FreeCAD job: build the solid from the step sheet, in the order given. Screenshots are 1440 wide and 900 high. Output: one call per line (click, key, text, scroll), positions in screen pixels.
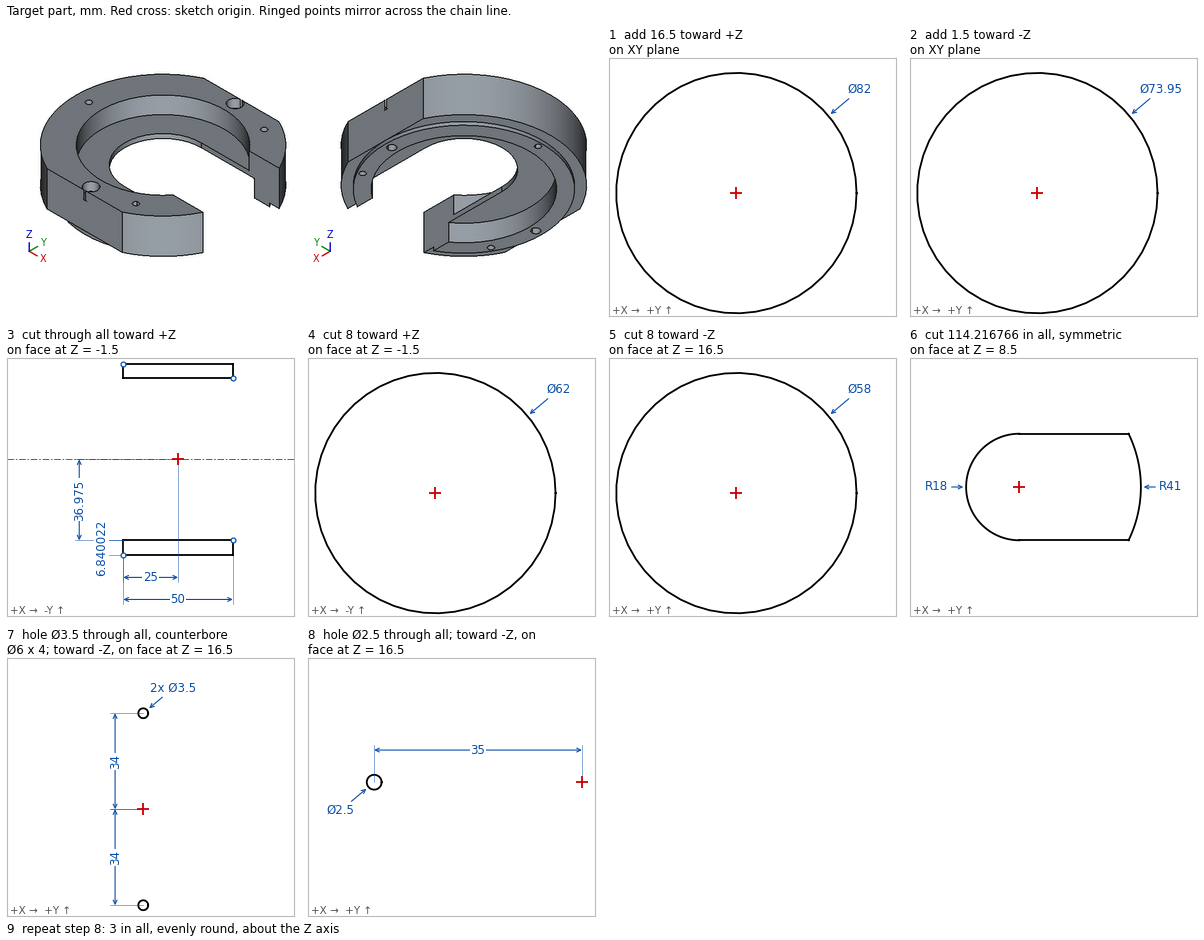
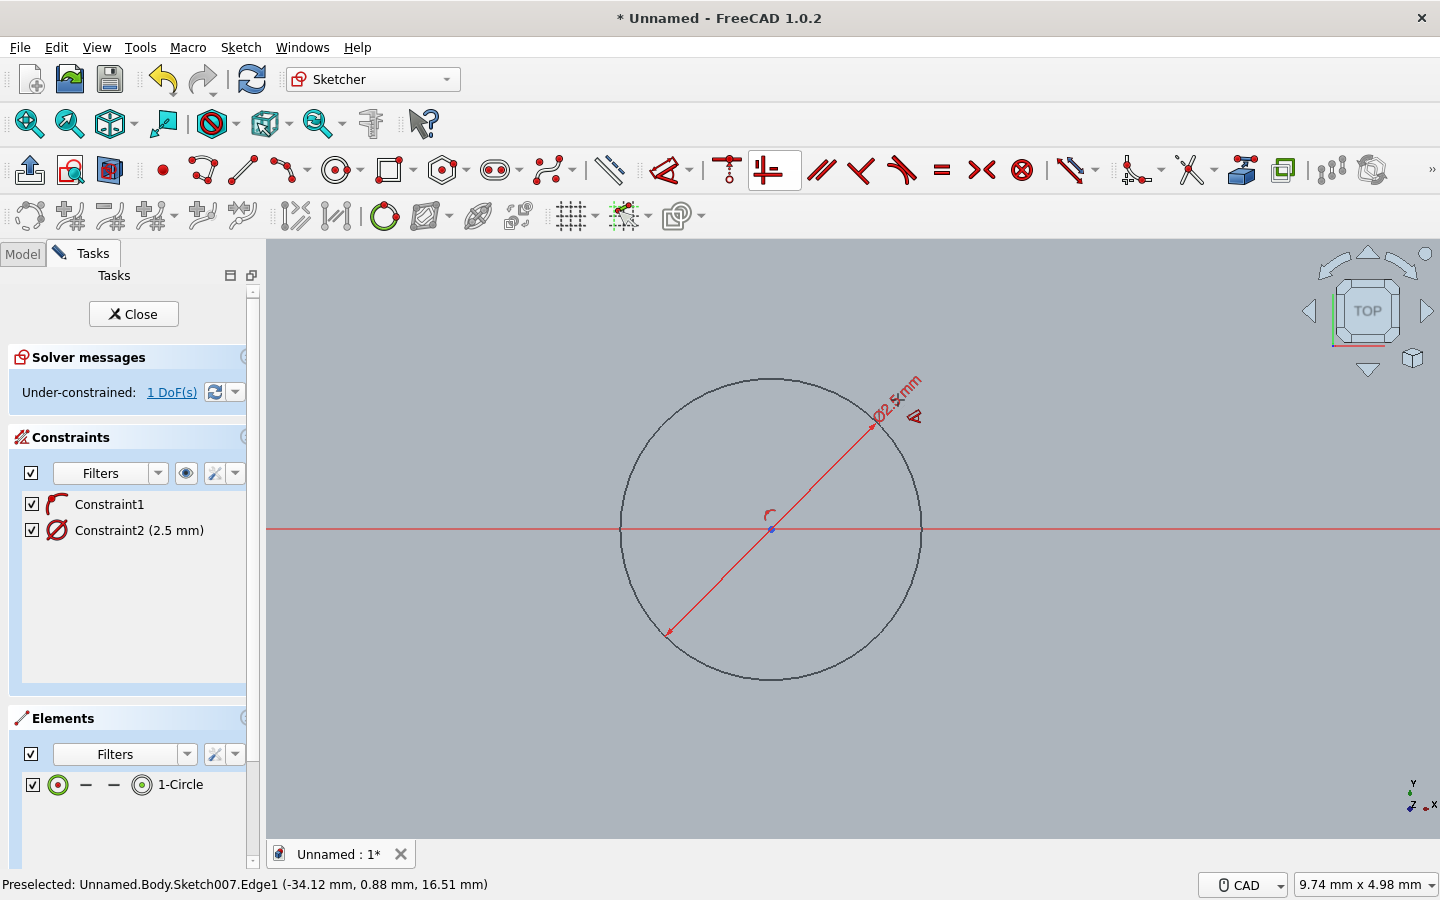
click(771, 529)
click(1023, 563)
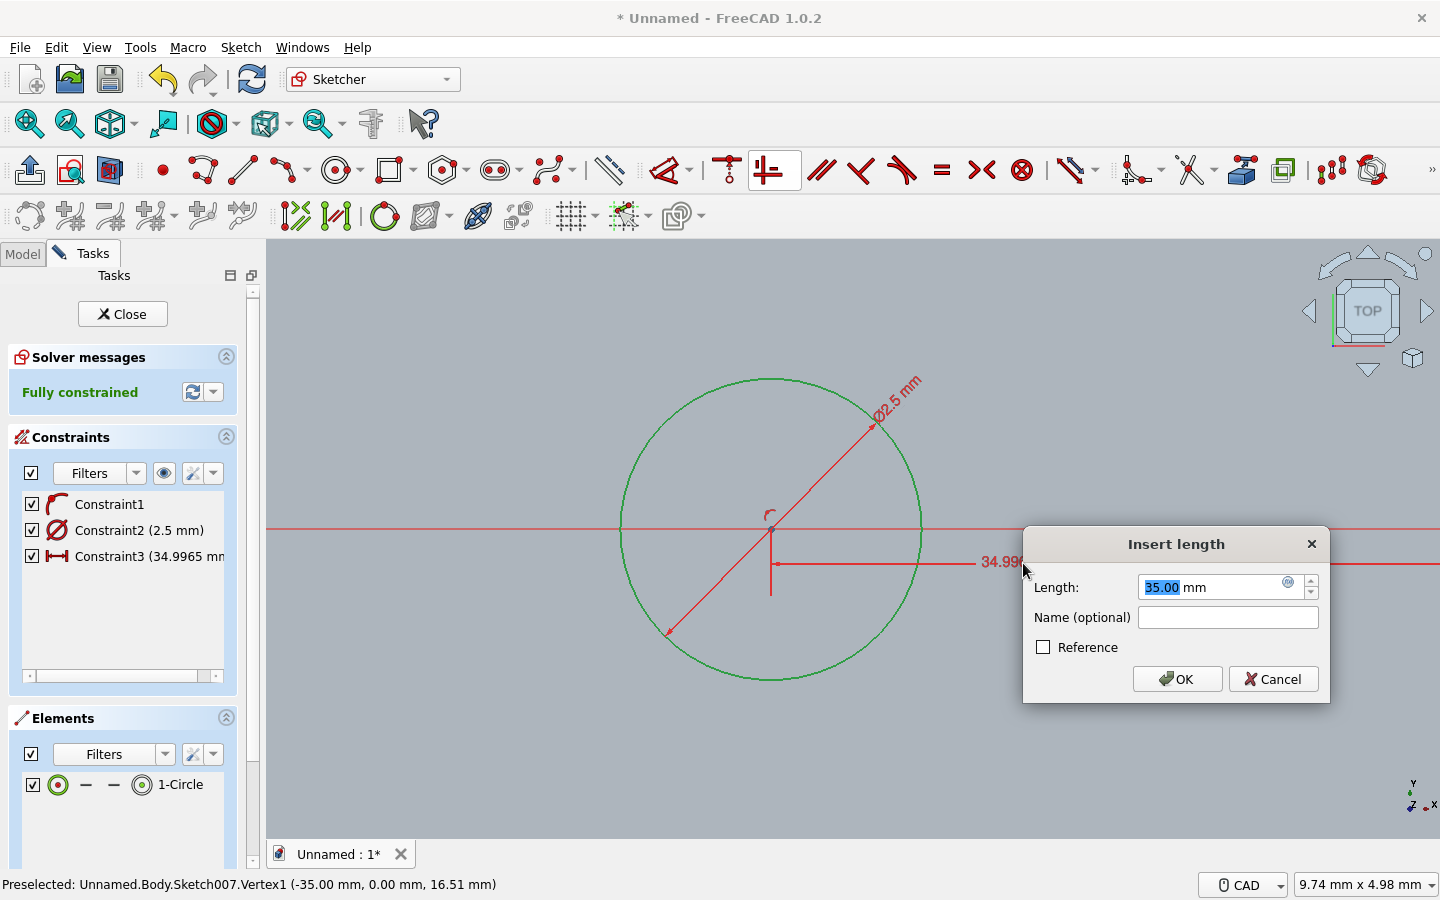
text(35)
key(Return)
key(Escape)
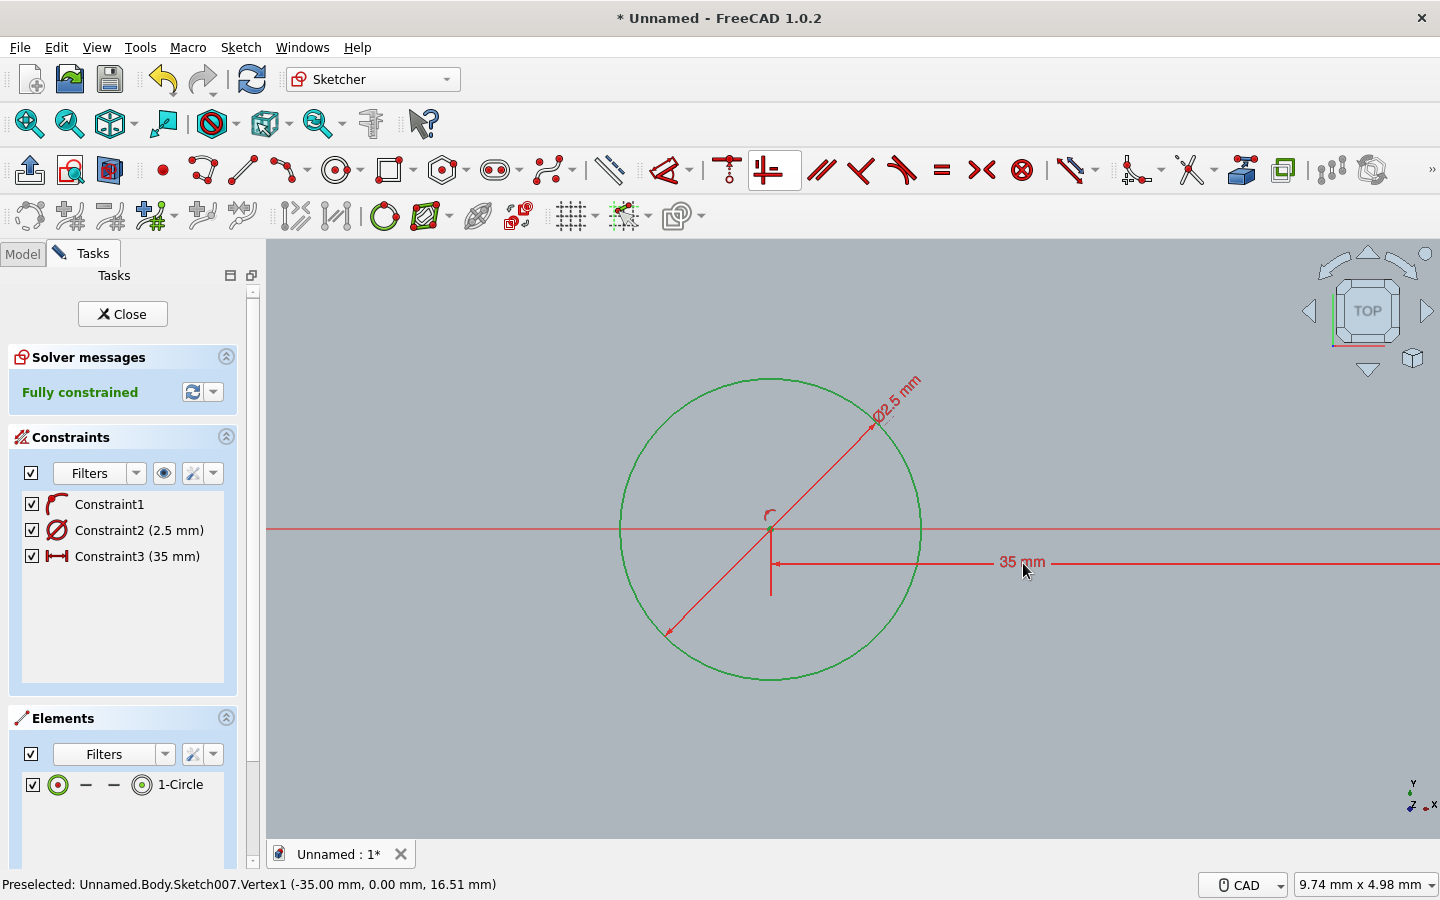
click(123, 314)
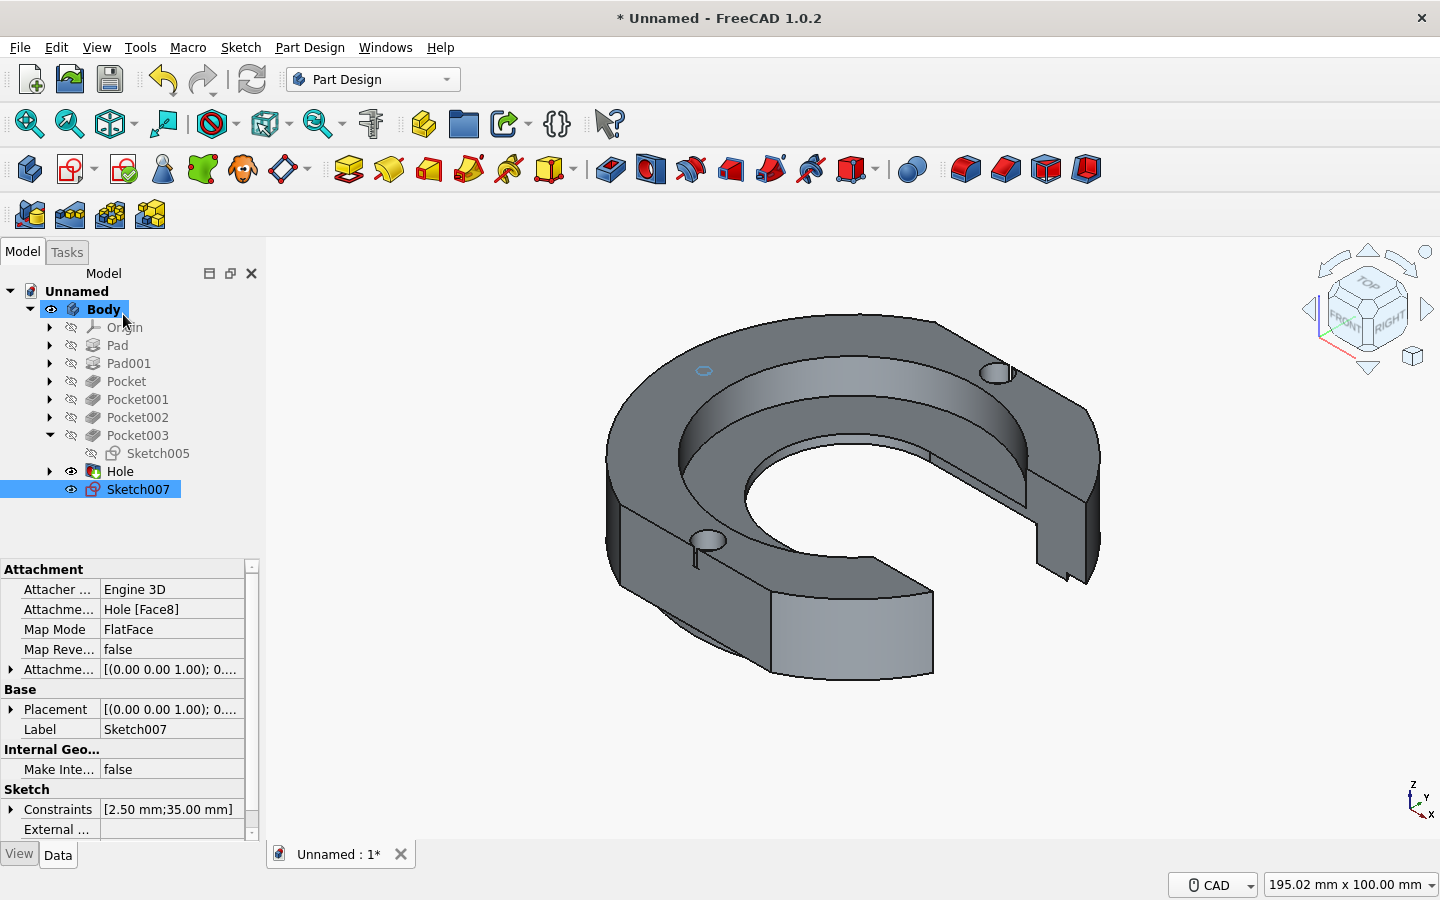
click(652, 170)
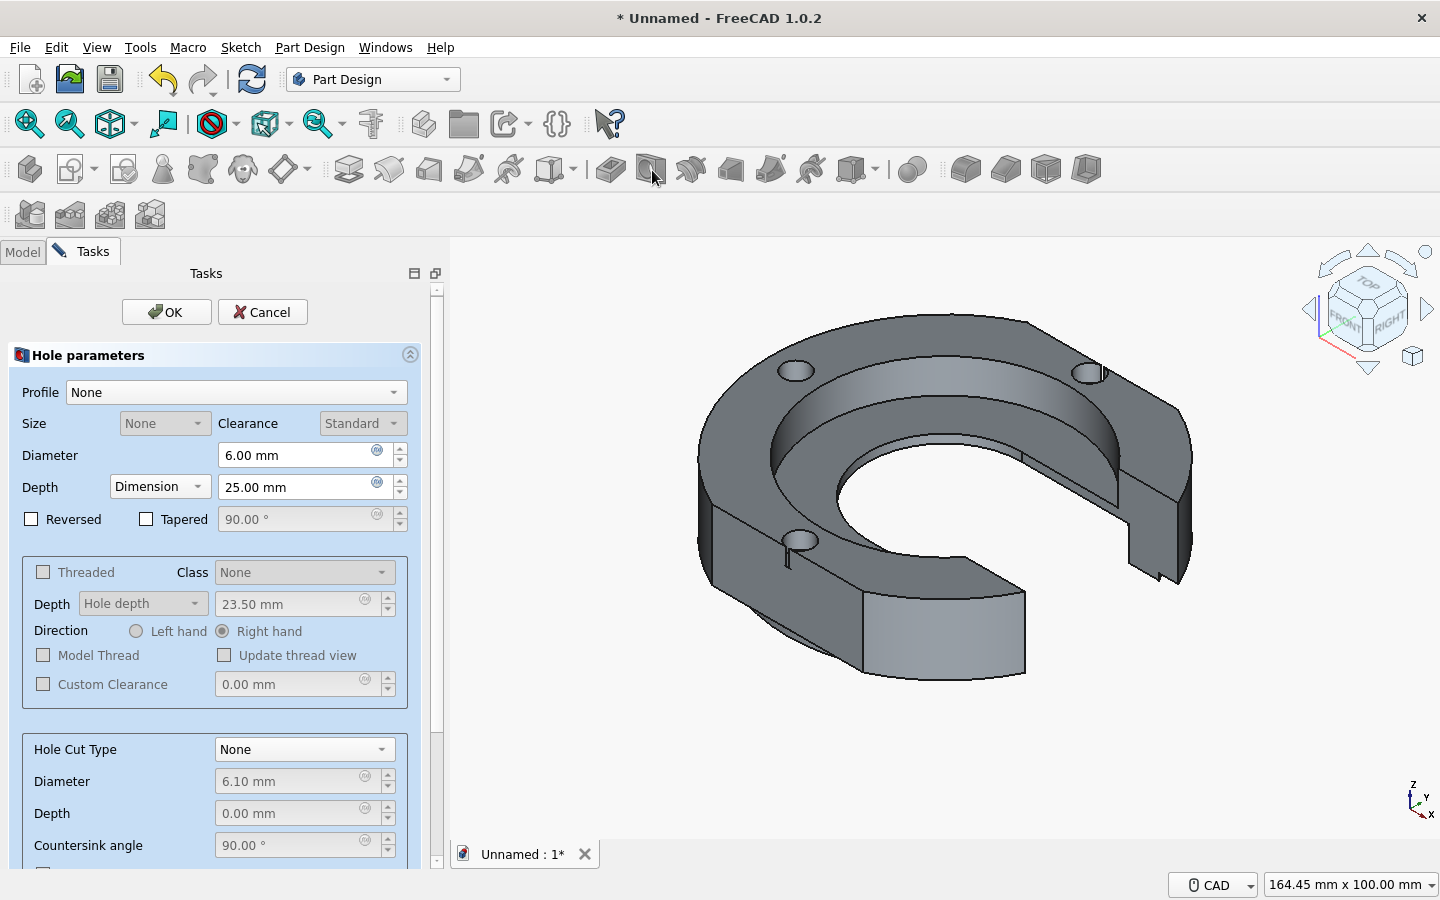
triple_click(305, 455)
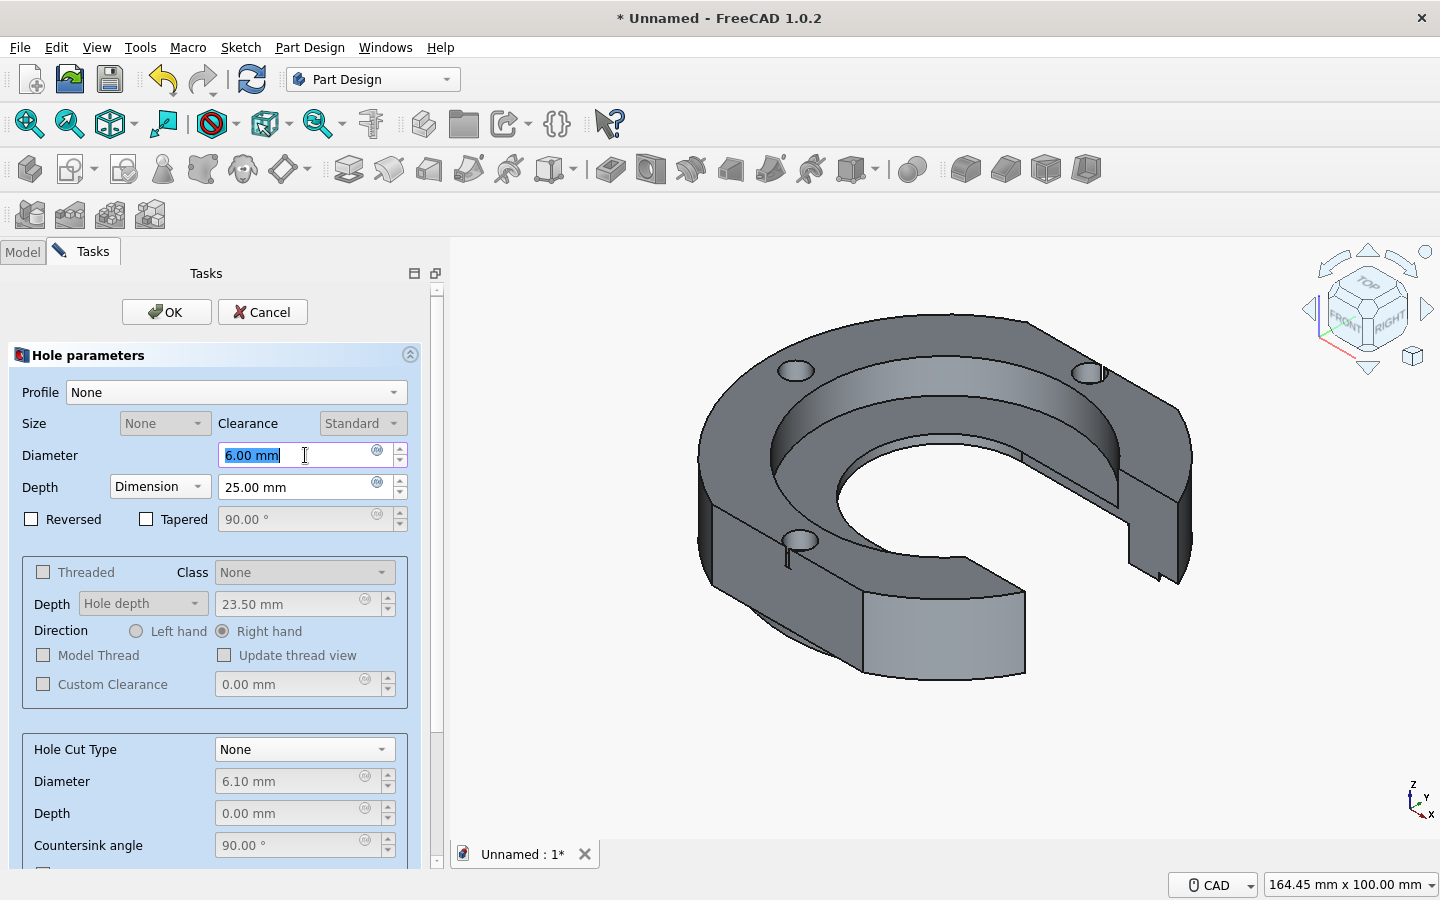
text(2.5)
key(Tab)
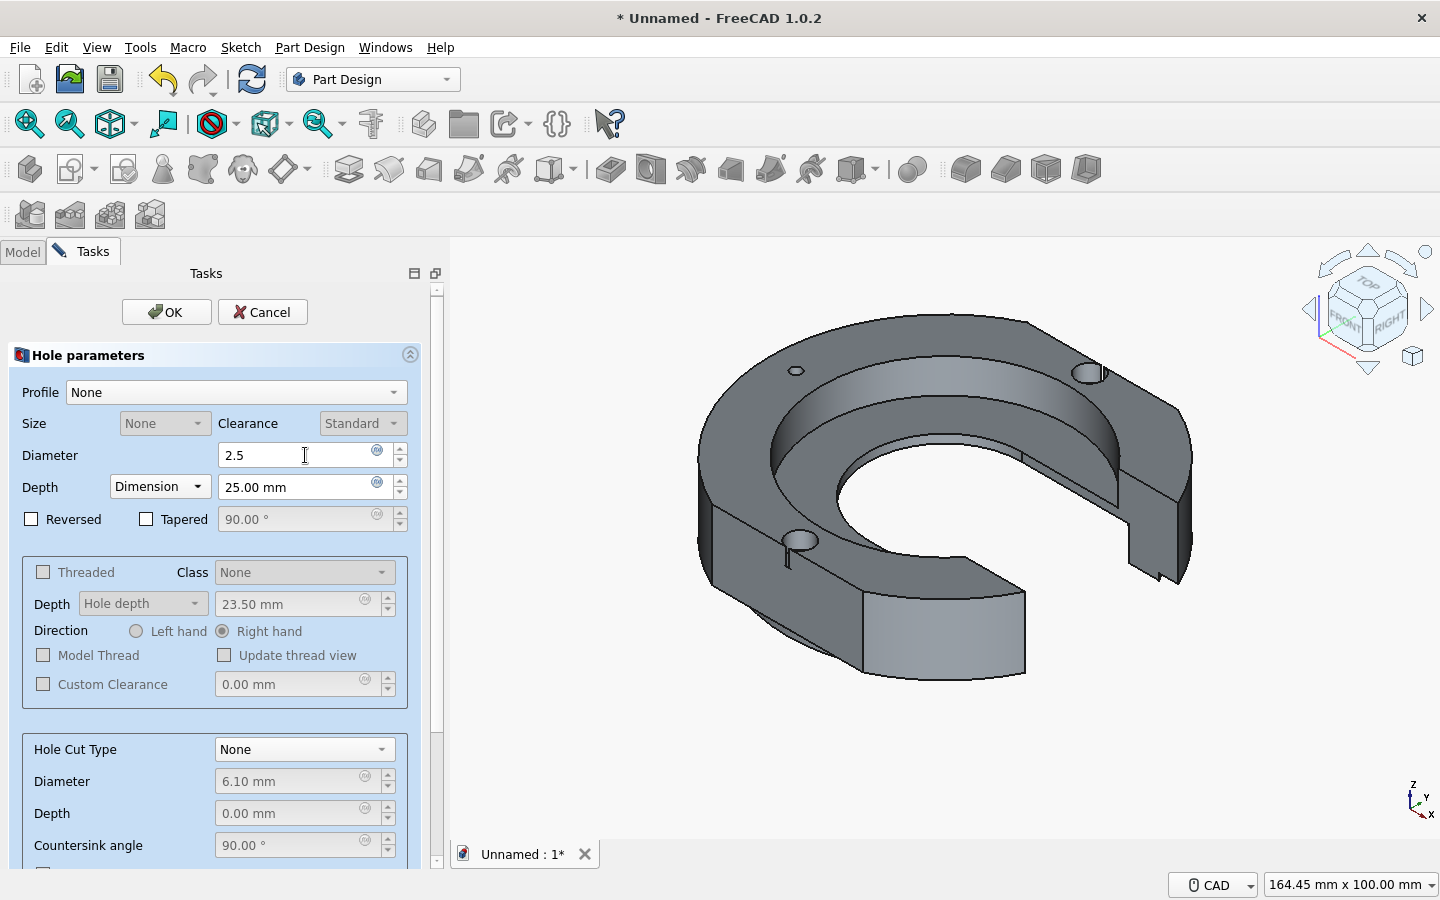
click(161, 486)